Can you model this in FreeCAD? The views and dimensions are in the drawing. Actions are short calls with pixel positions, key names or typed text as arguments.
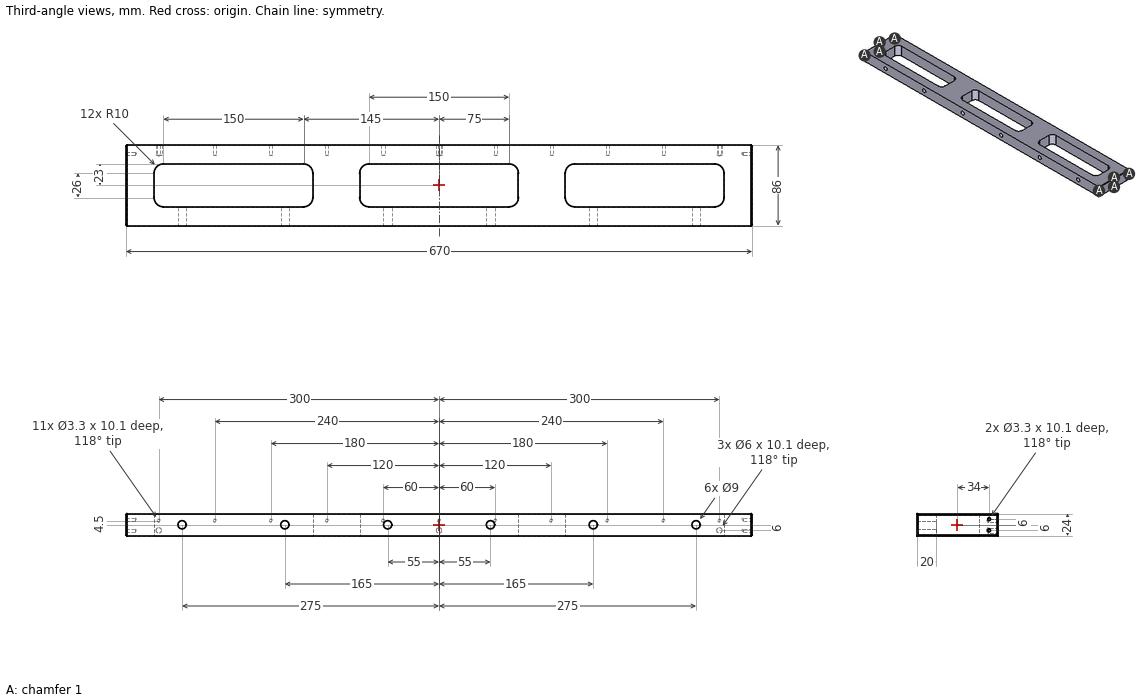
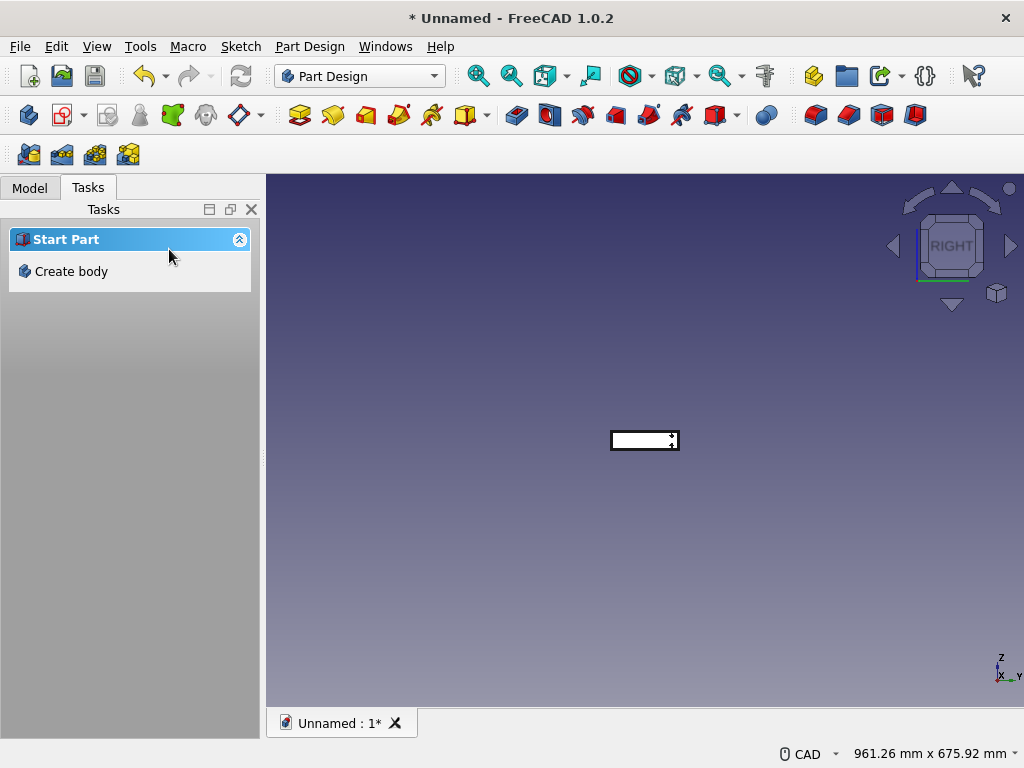
key(0)